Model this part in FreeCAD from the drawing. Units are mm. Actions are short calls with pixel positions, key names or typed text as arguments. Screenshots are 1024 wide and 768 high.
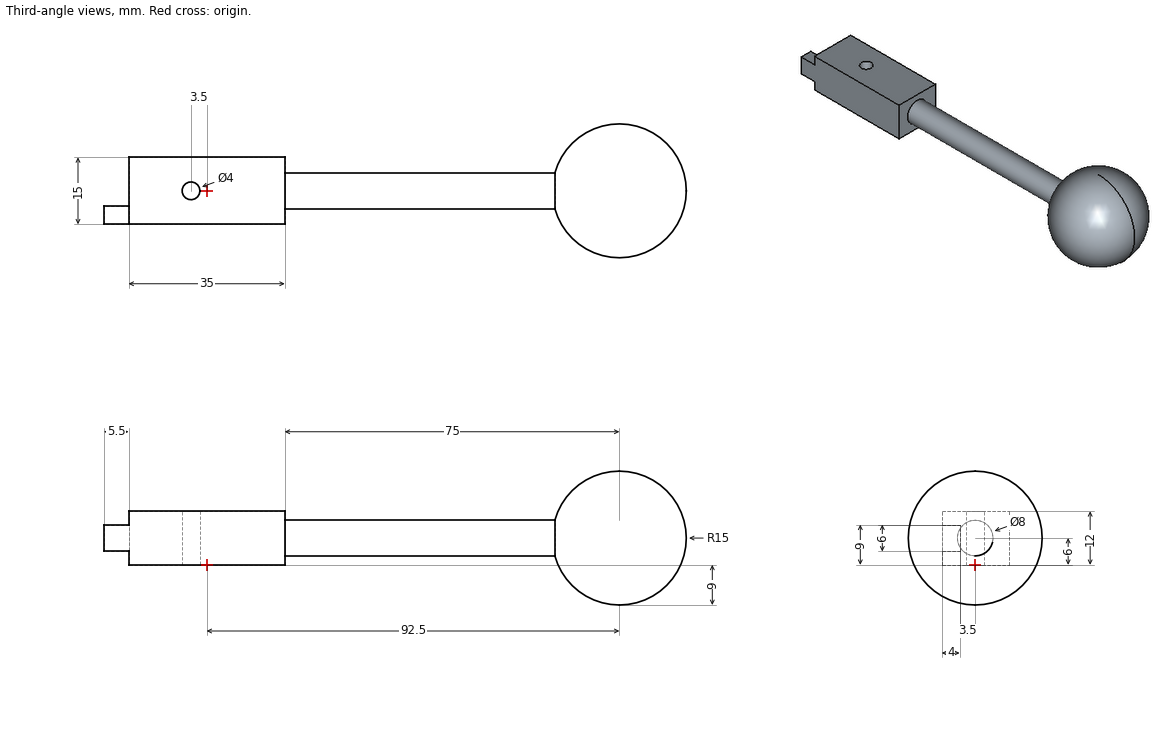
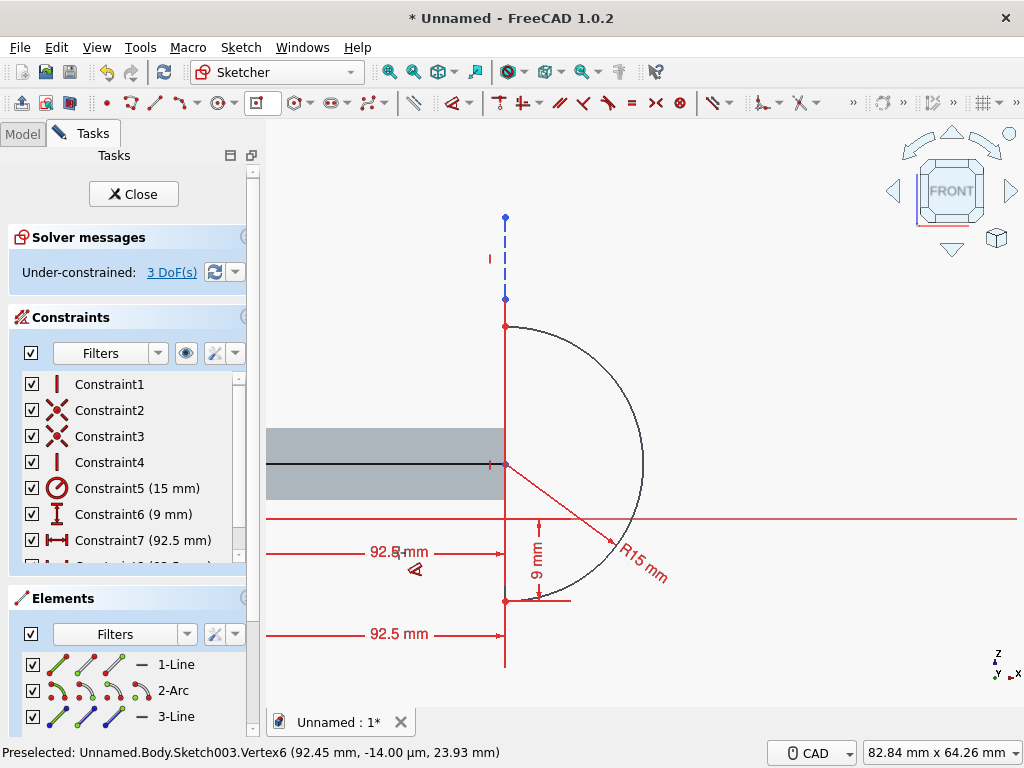
click(506, 464)
click(326, 553)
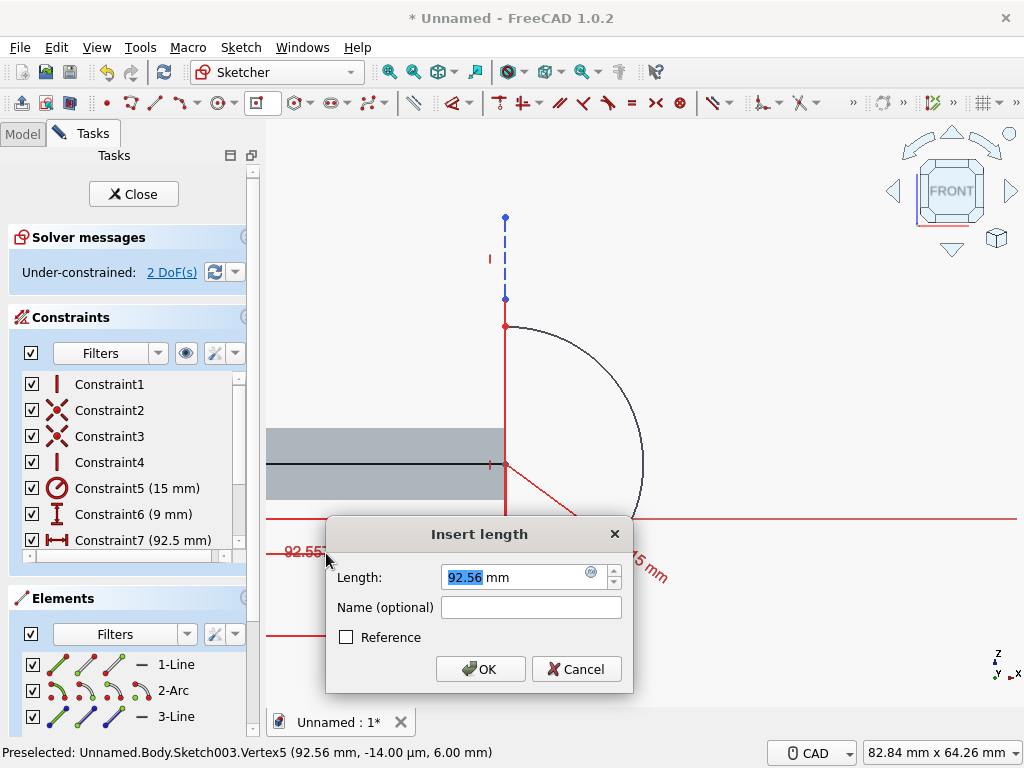
text(92.5)
key(Return)
key(Escape)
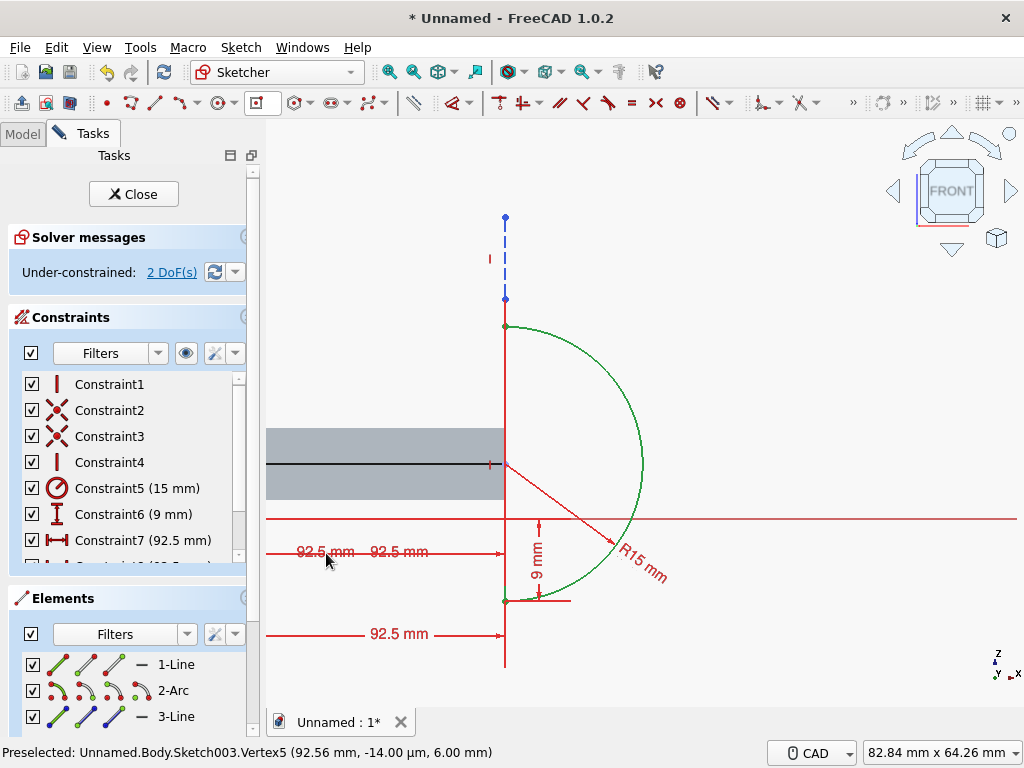
click(134, 194)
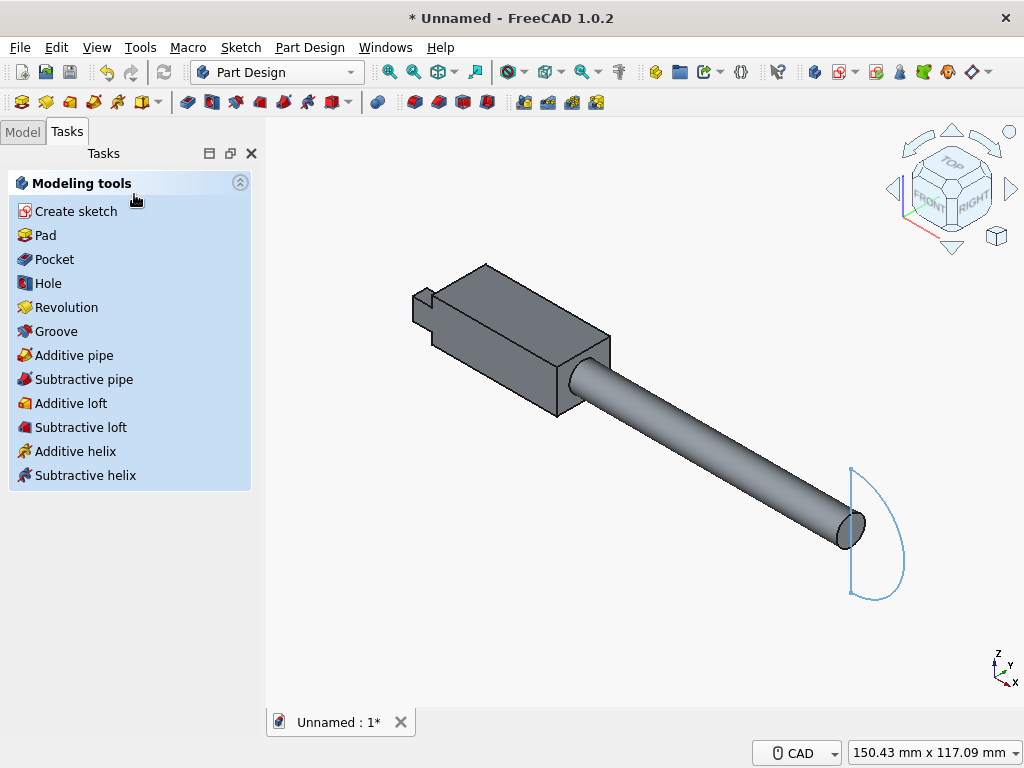
click(46, 102)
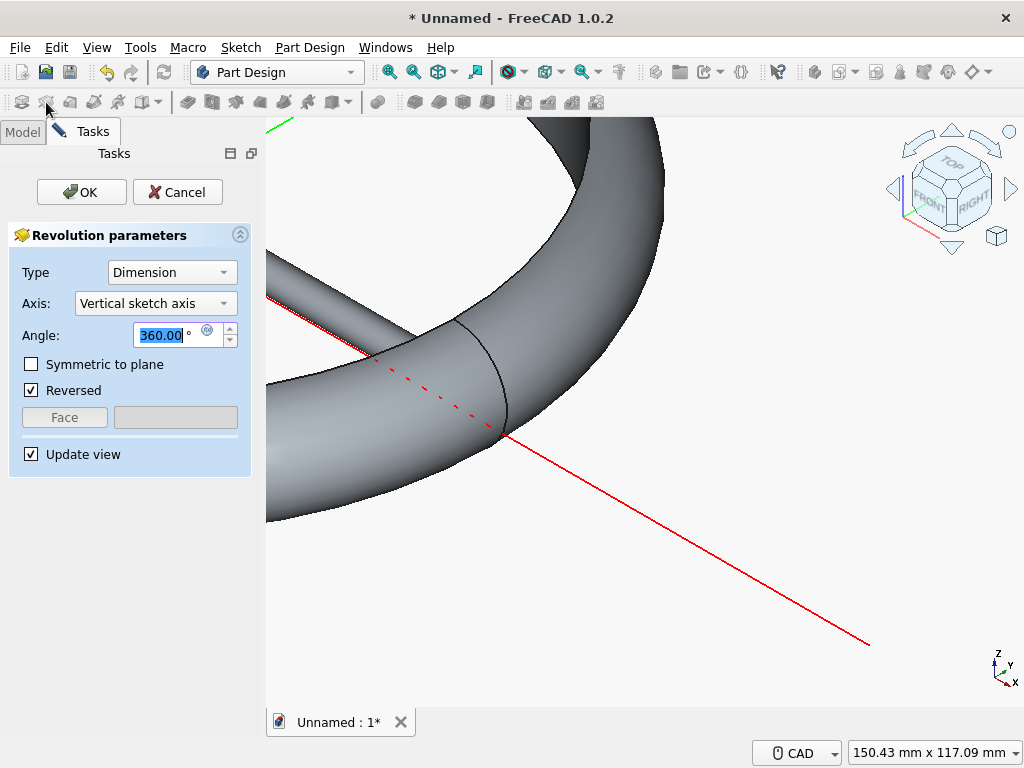
click(156, 304)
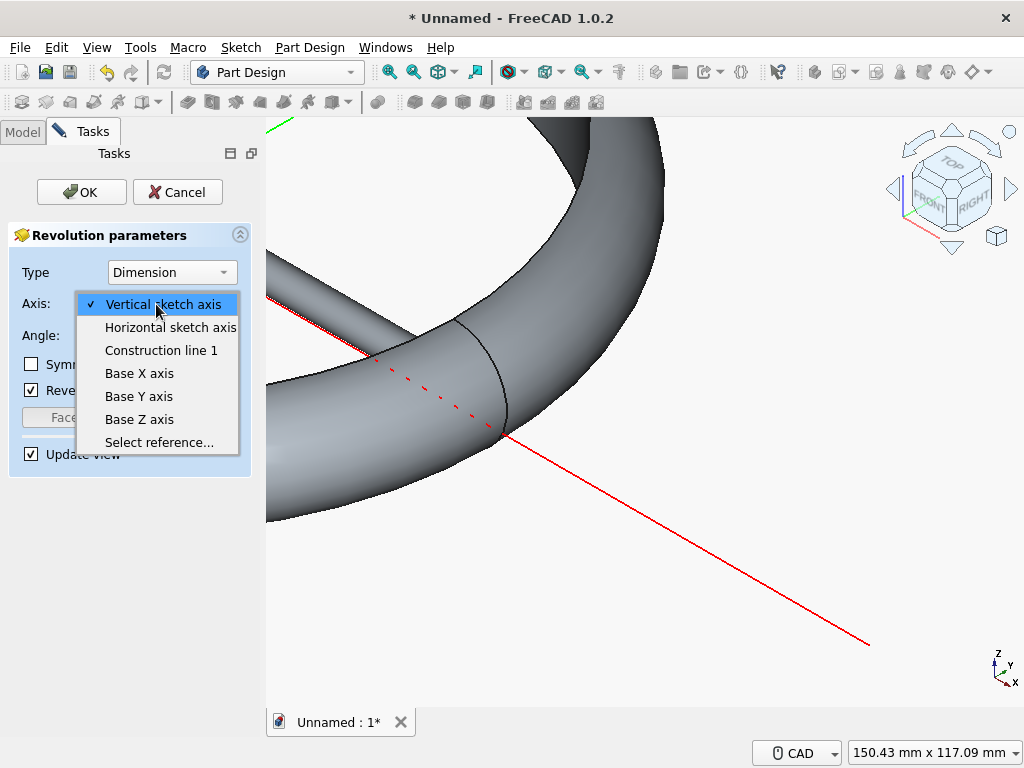
click(156, 350)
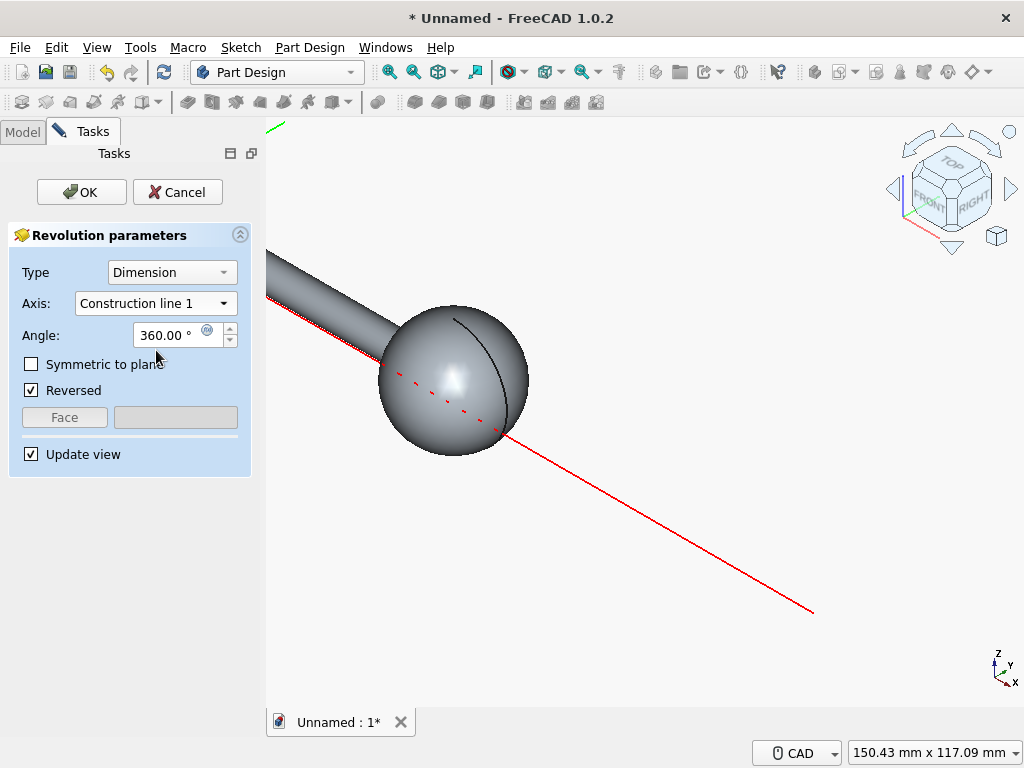
click(82, 192)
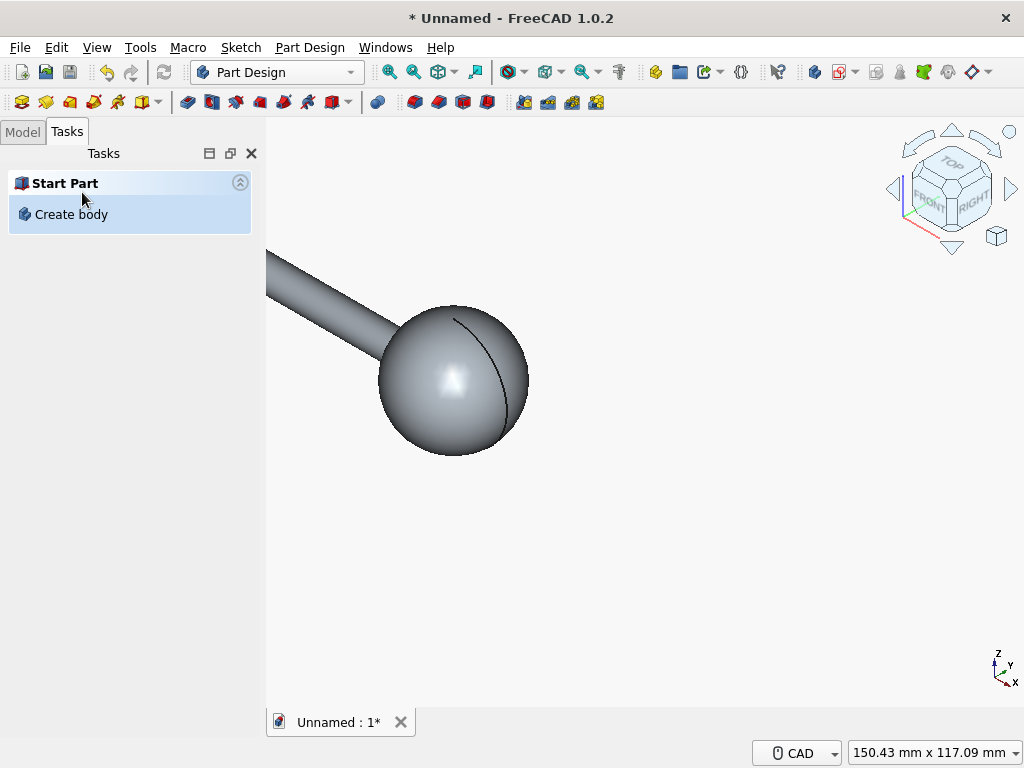
key(v)
key(f)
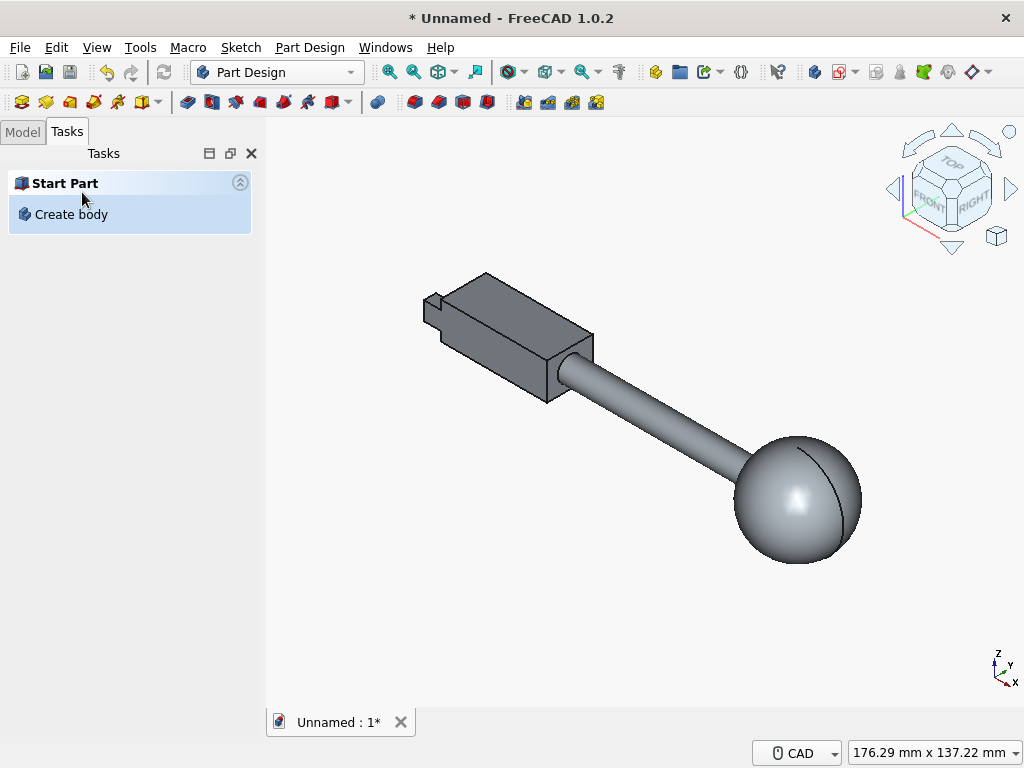
click(547, 333)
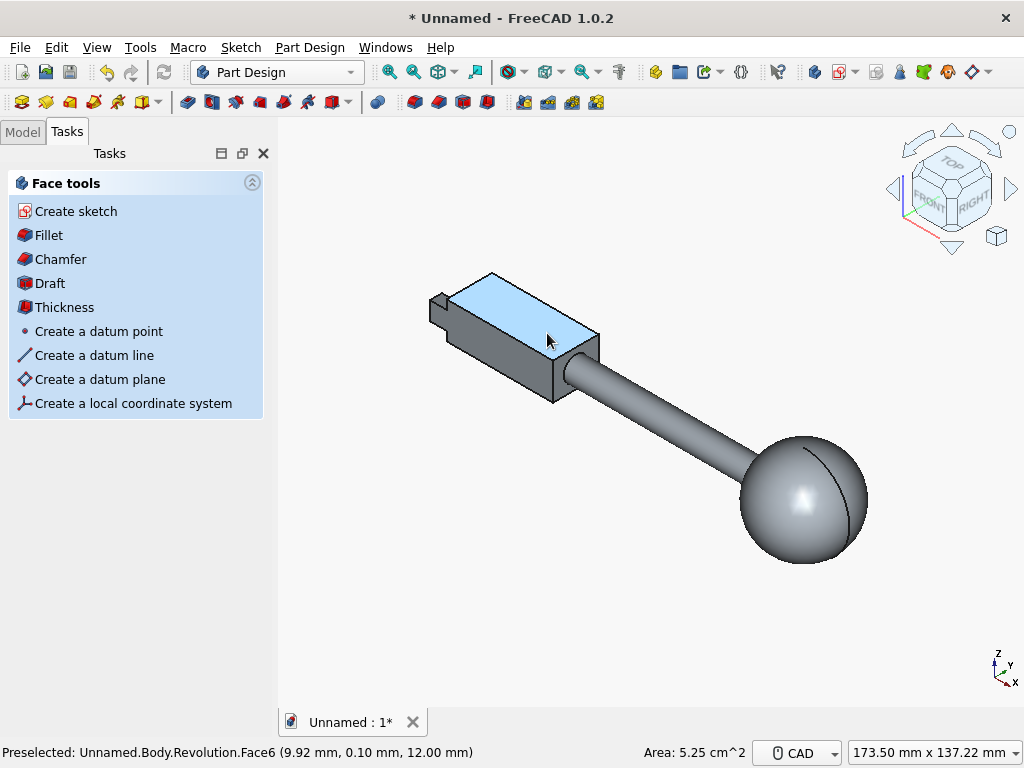
click(840, 72)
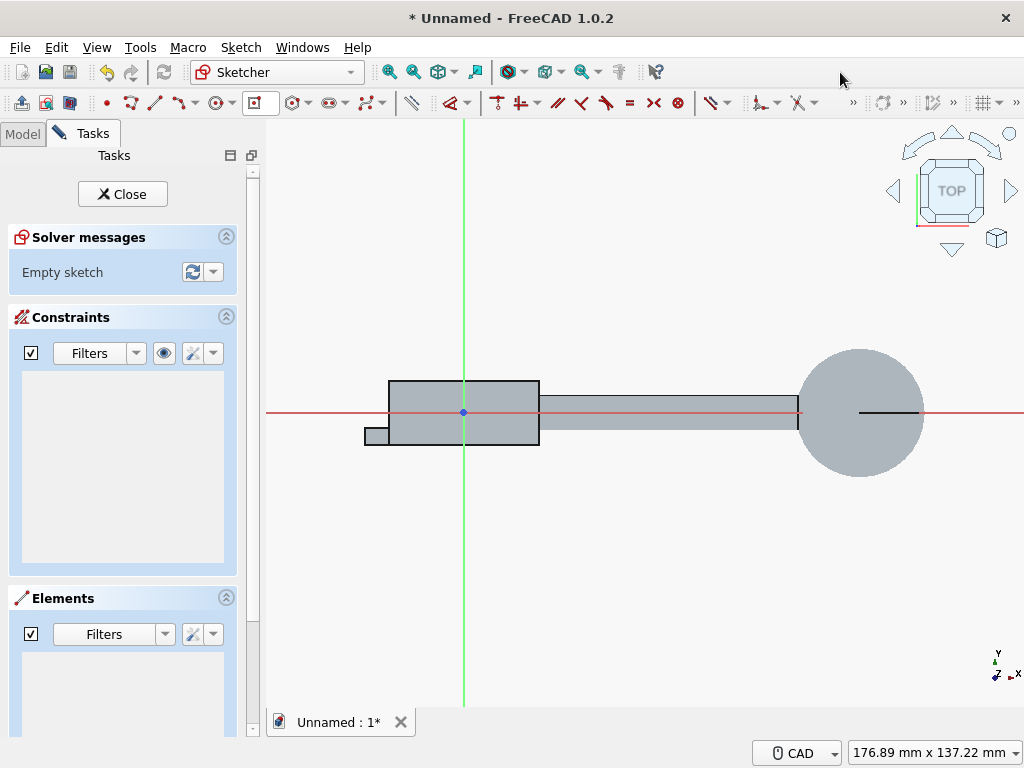
click(70, 104)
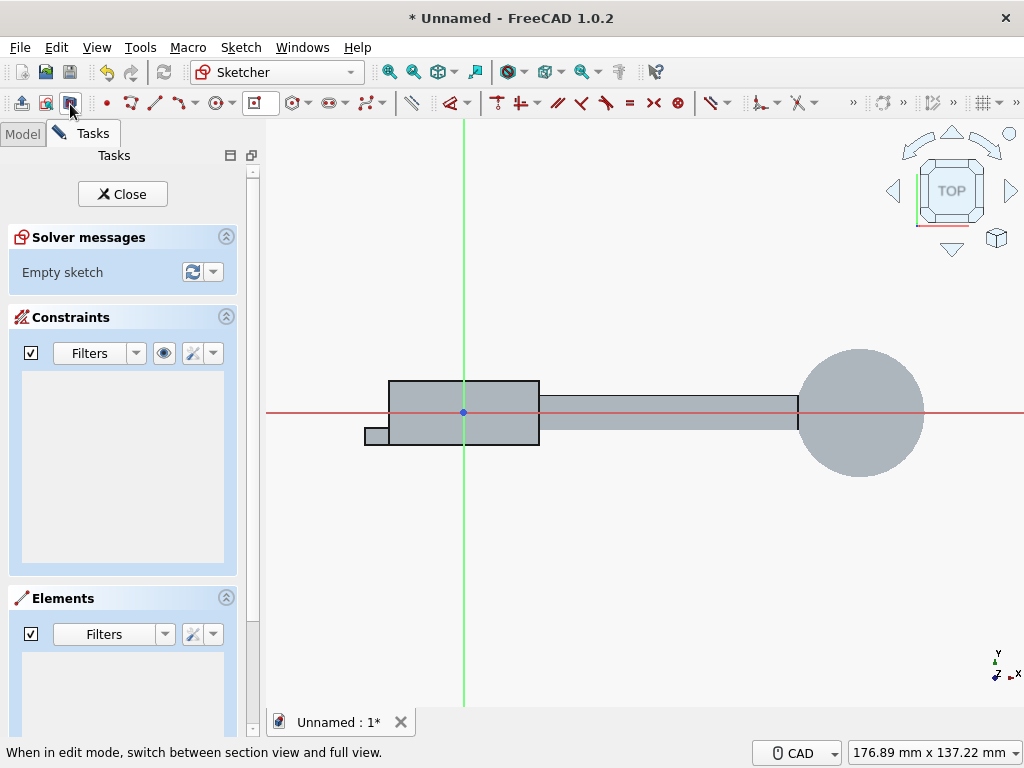
scroll(444, 413, up, 14)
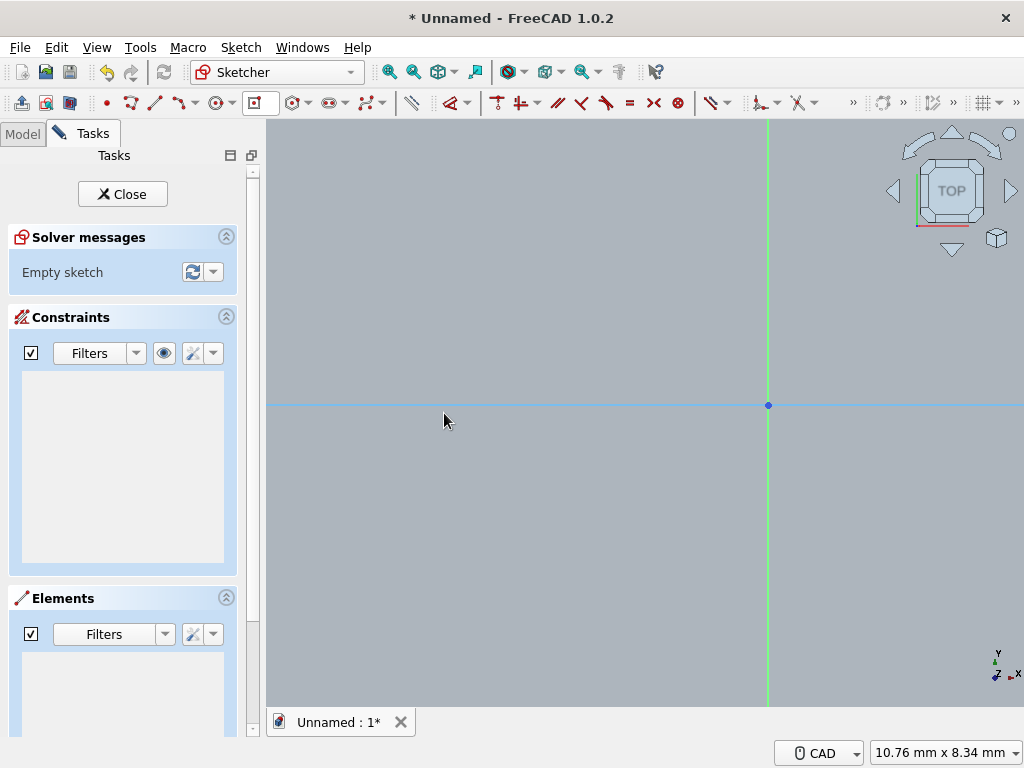
key(g)
key(c)